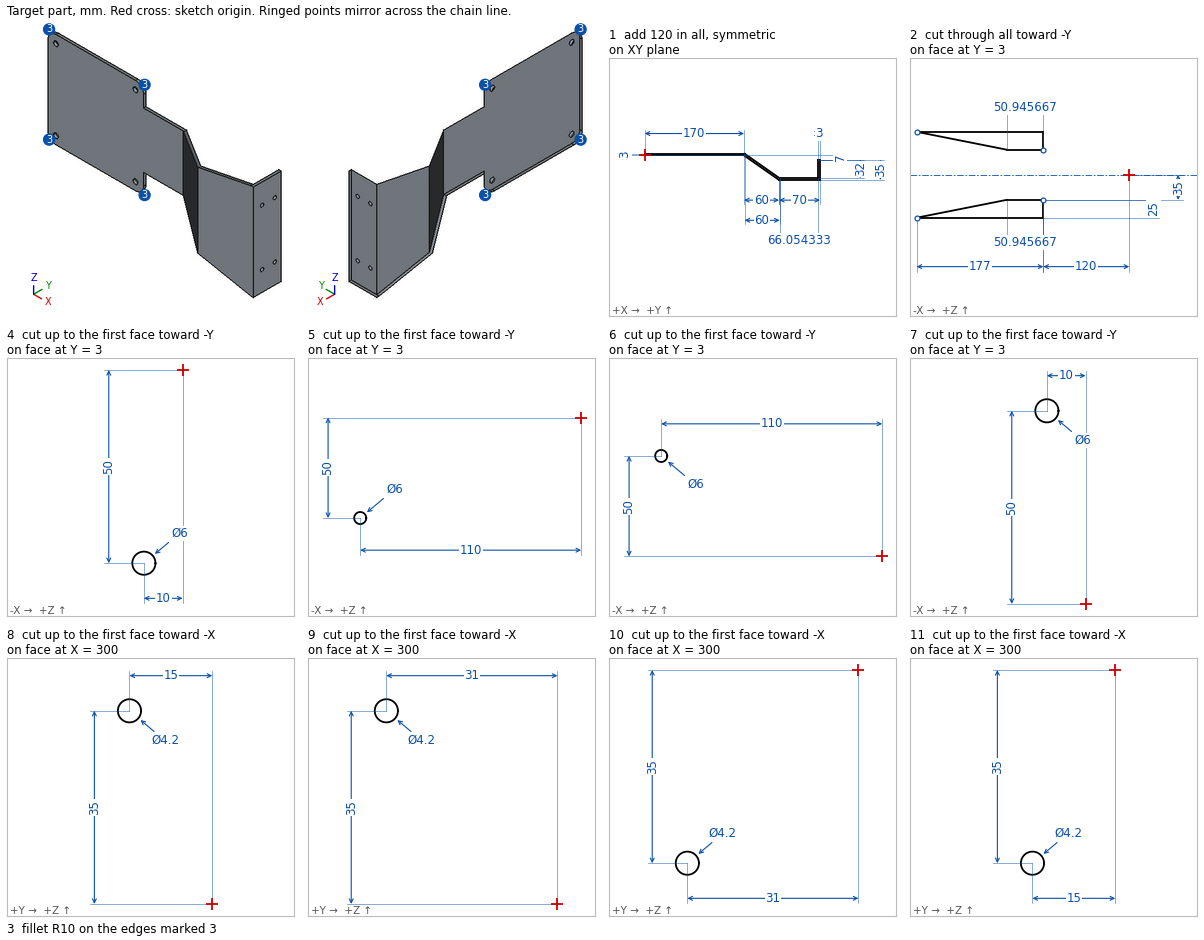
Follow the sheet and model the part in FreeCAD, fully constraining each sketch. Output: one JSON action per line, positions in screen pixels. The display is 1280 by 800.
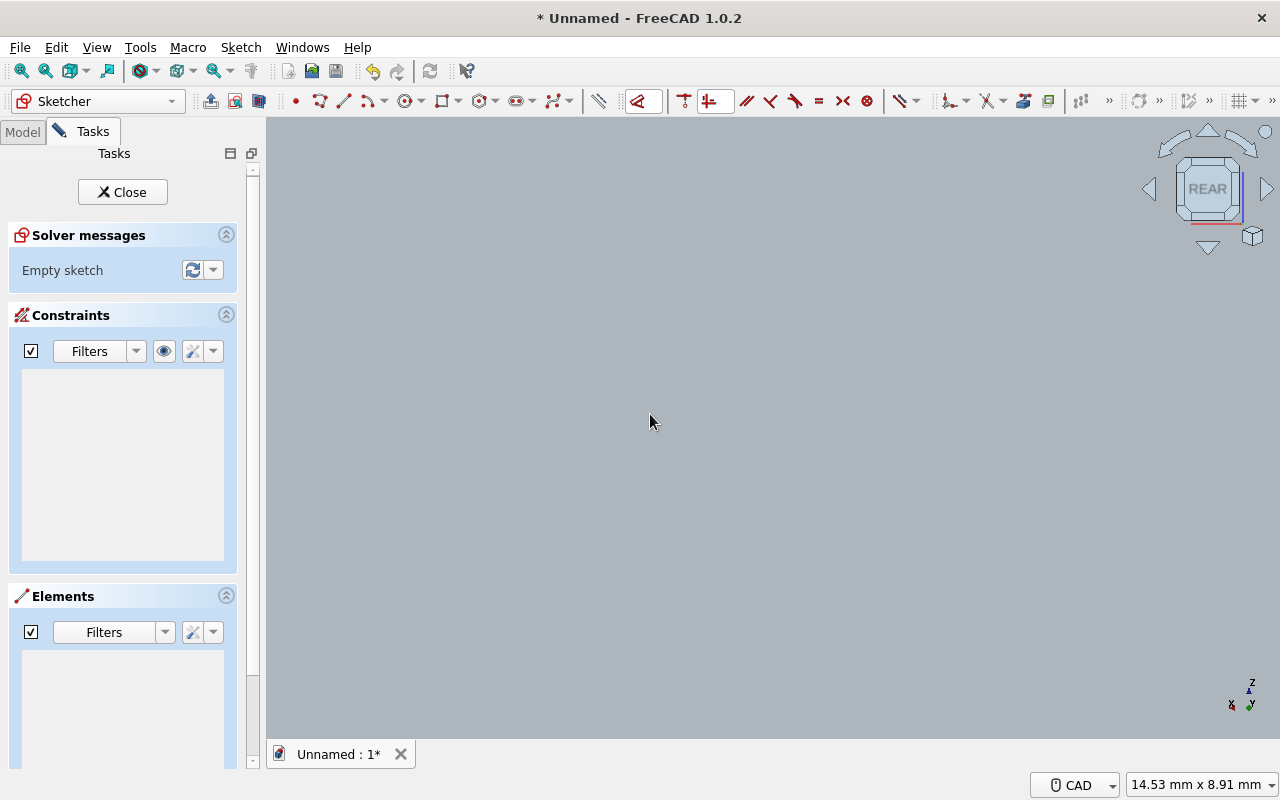
{"action": "left_click", "coordinate": [406, 102]}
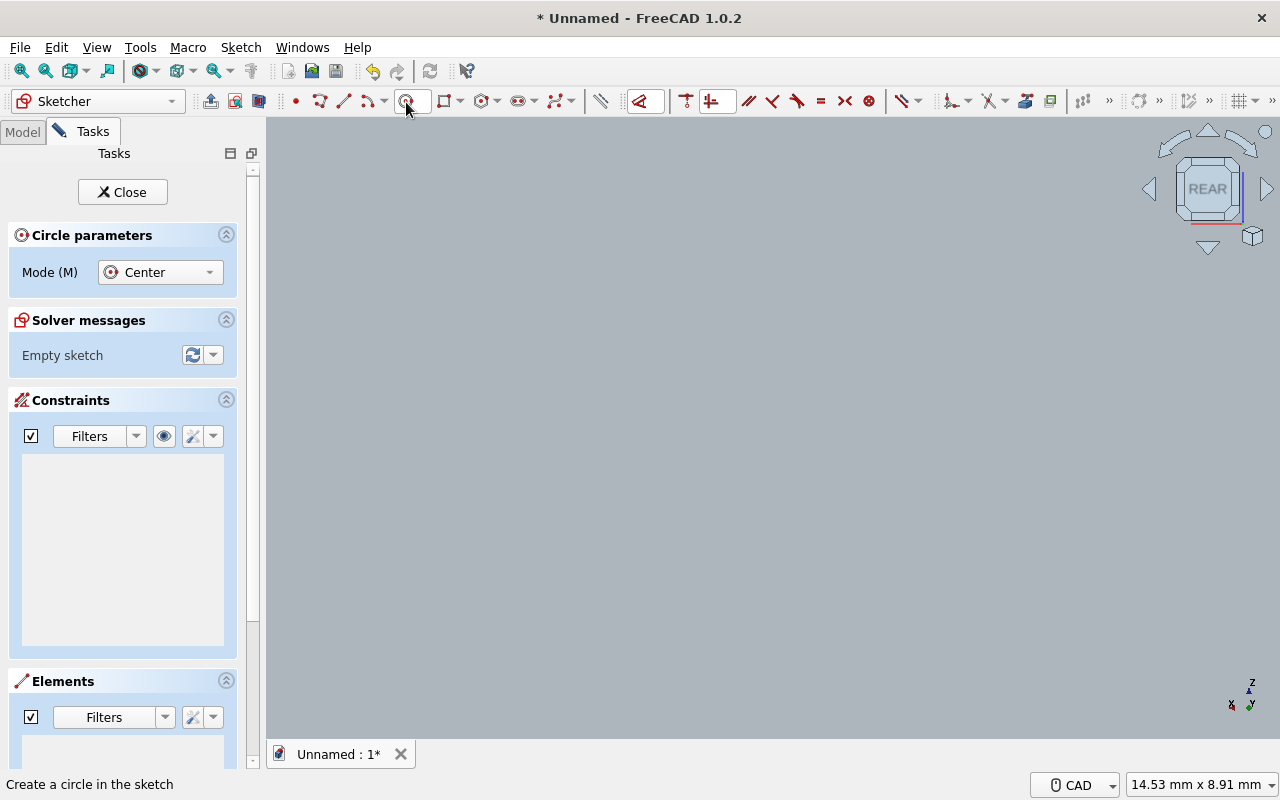
{"action": "left_click", "coordinate": [705, 427]}
{"action": "left_click", "coordinate": [853, 279]}
{"action": "key", "text": "Escape"}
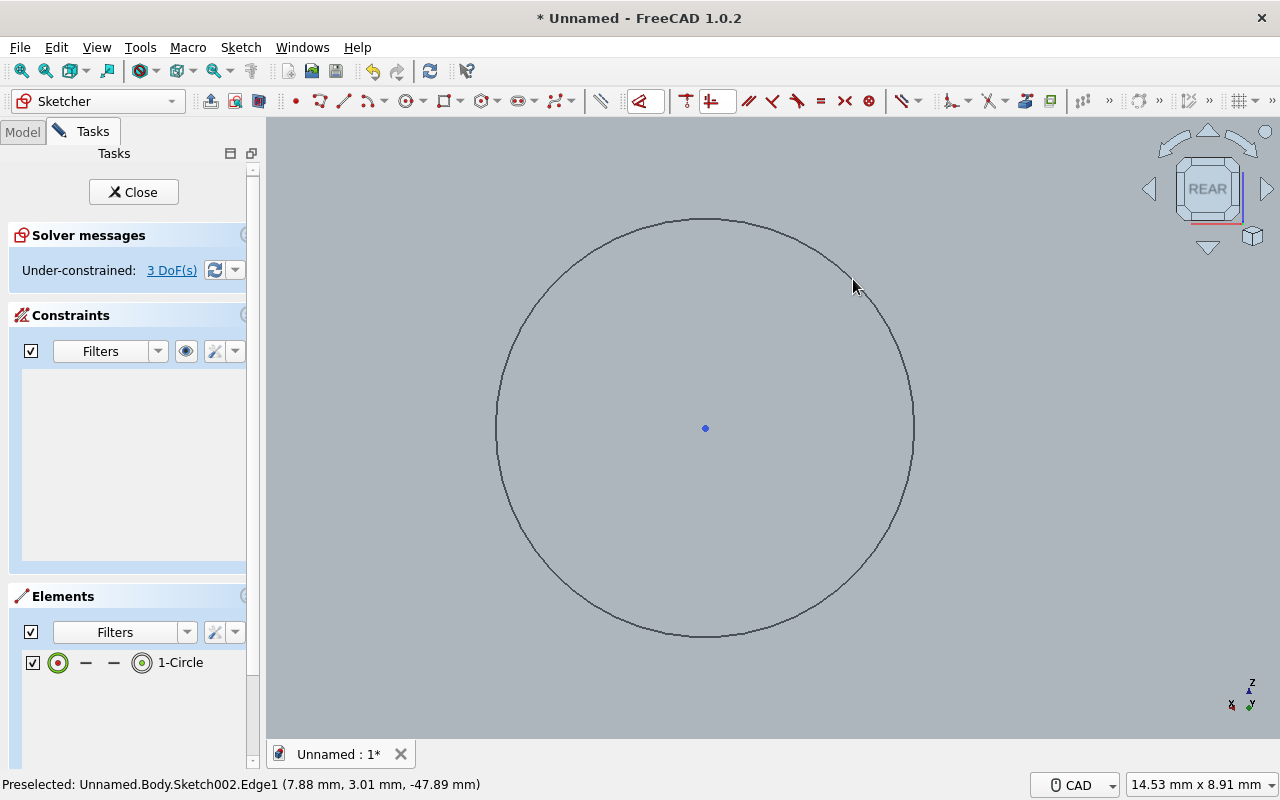
{"action": "left_click", "coordinate": [853, 280]}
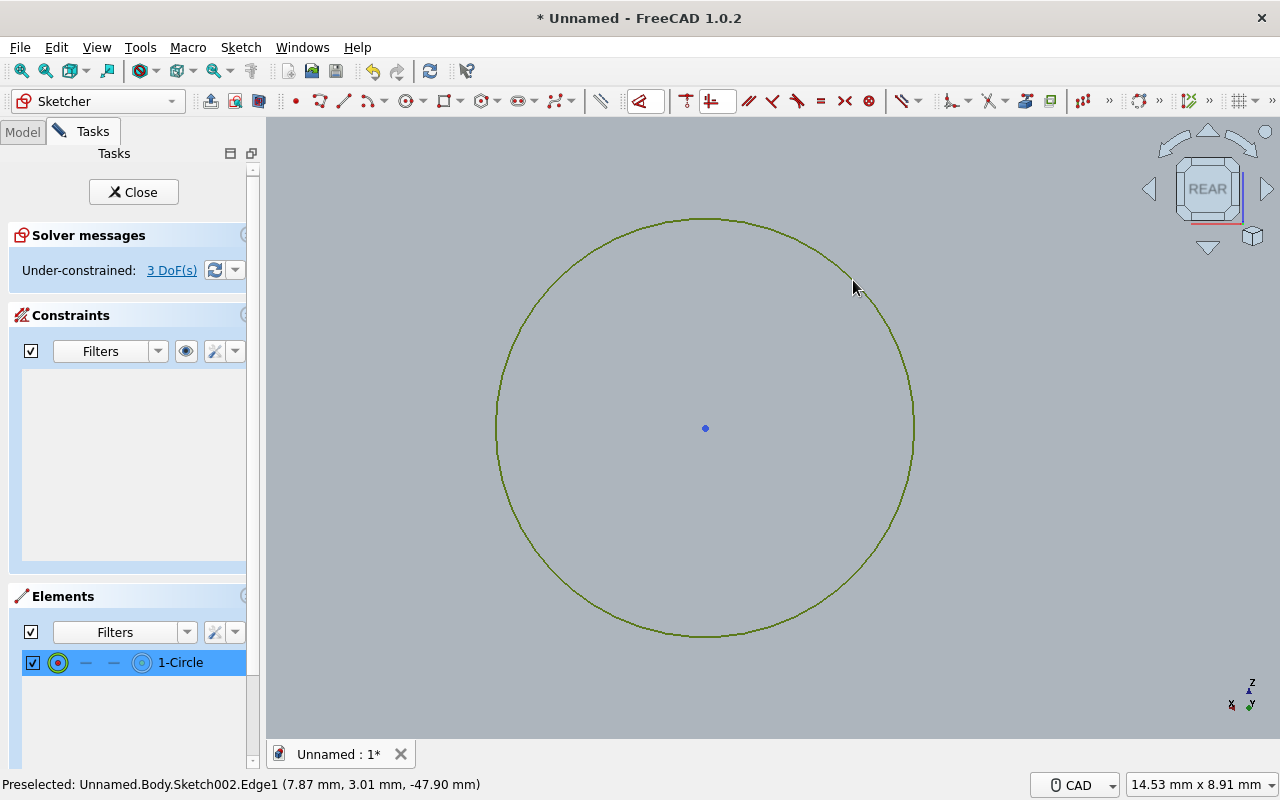
{"action": "key", "text": "k o"}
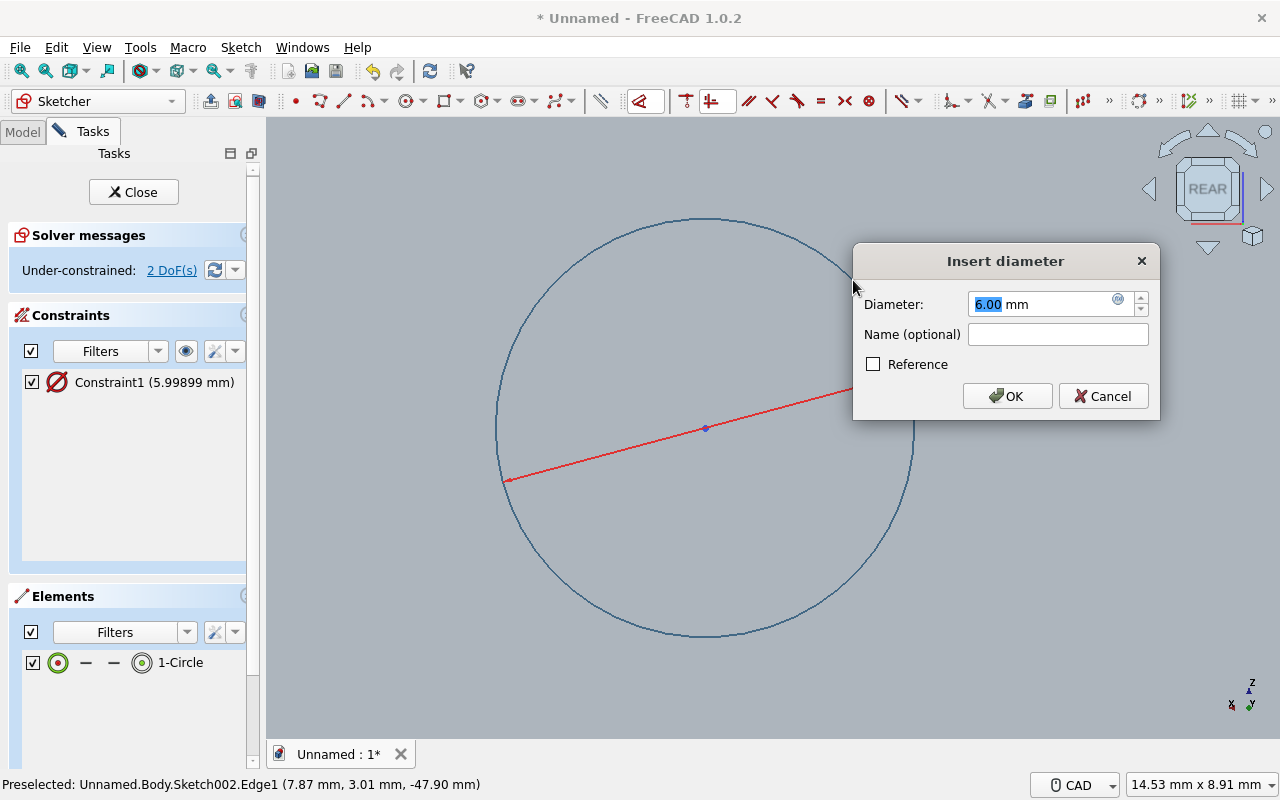
{"action": "type", "text": "6"}
{"action": "key", "text": "Return"}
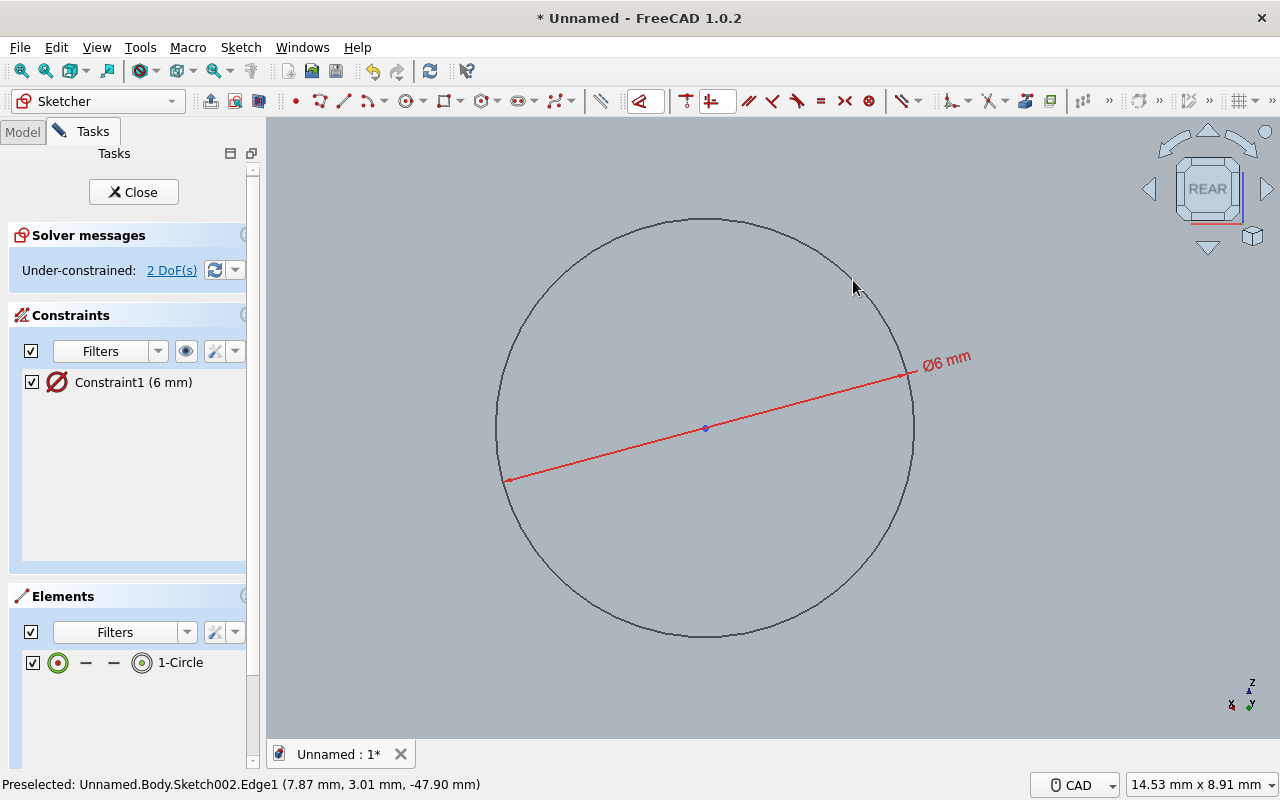
{"action": "left_click", "coordinate": [705, 428]}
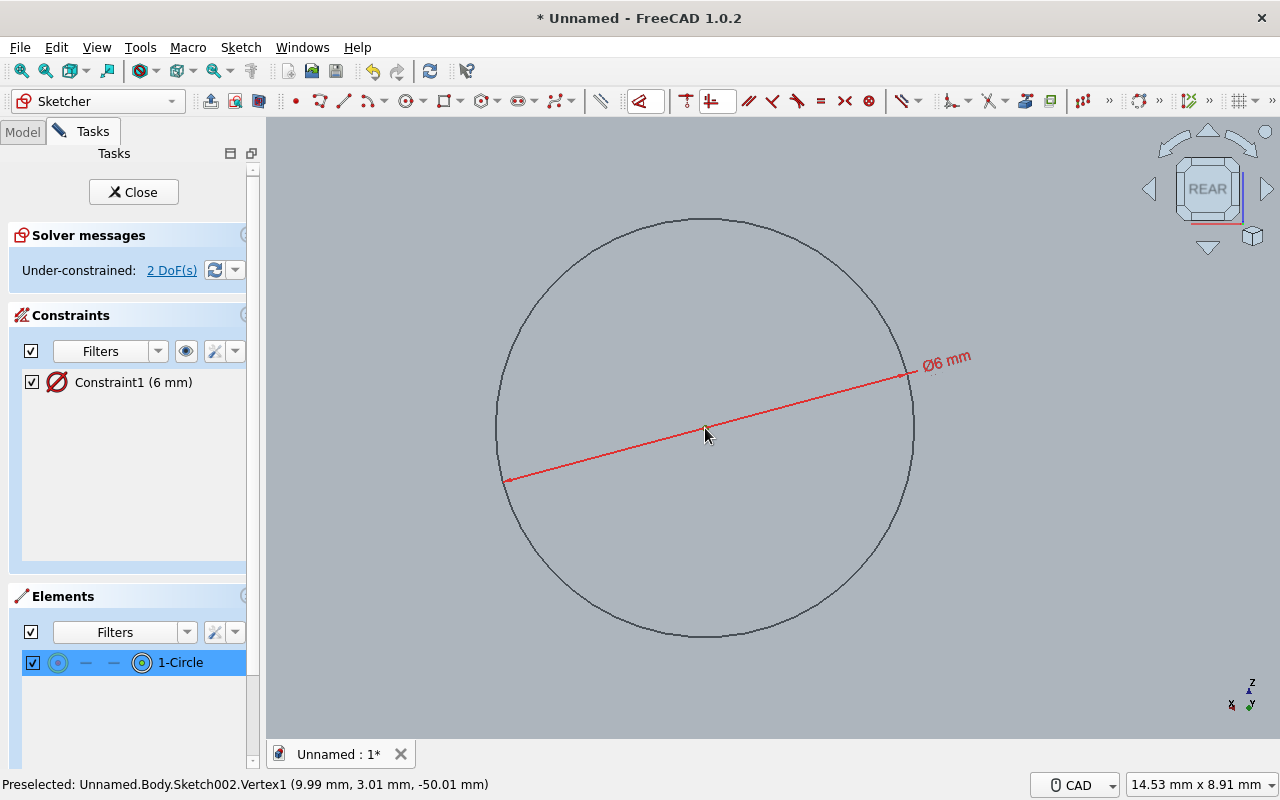
{"action": "key", "text": "l"}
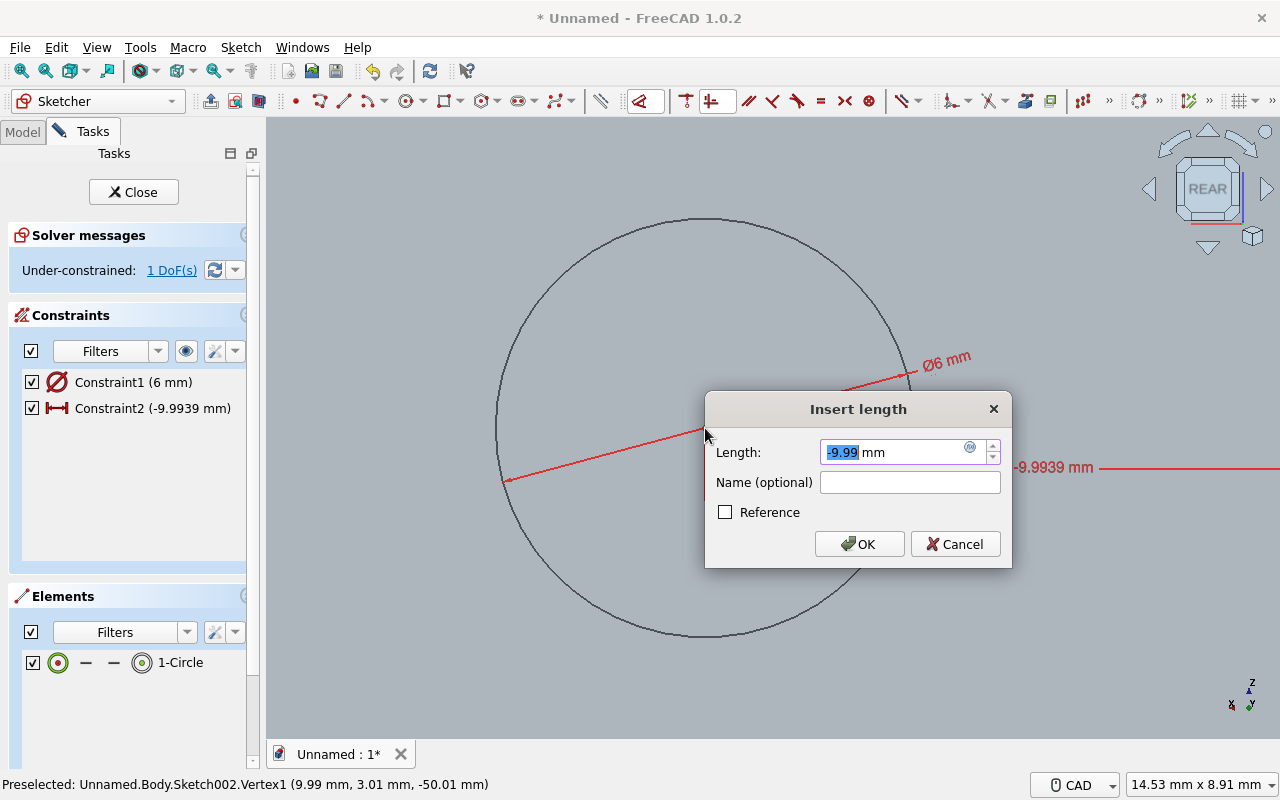
{"action": "type", "text": "-10"}
{"action": "key", "text": "Return"}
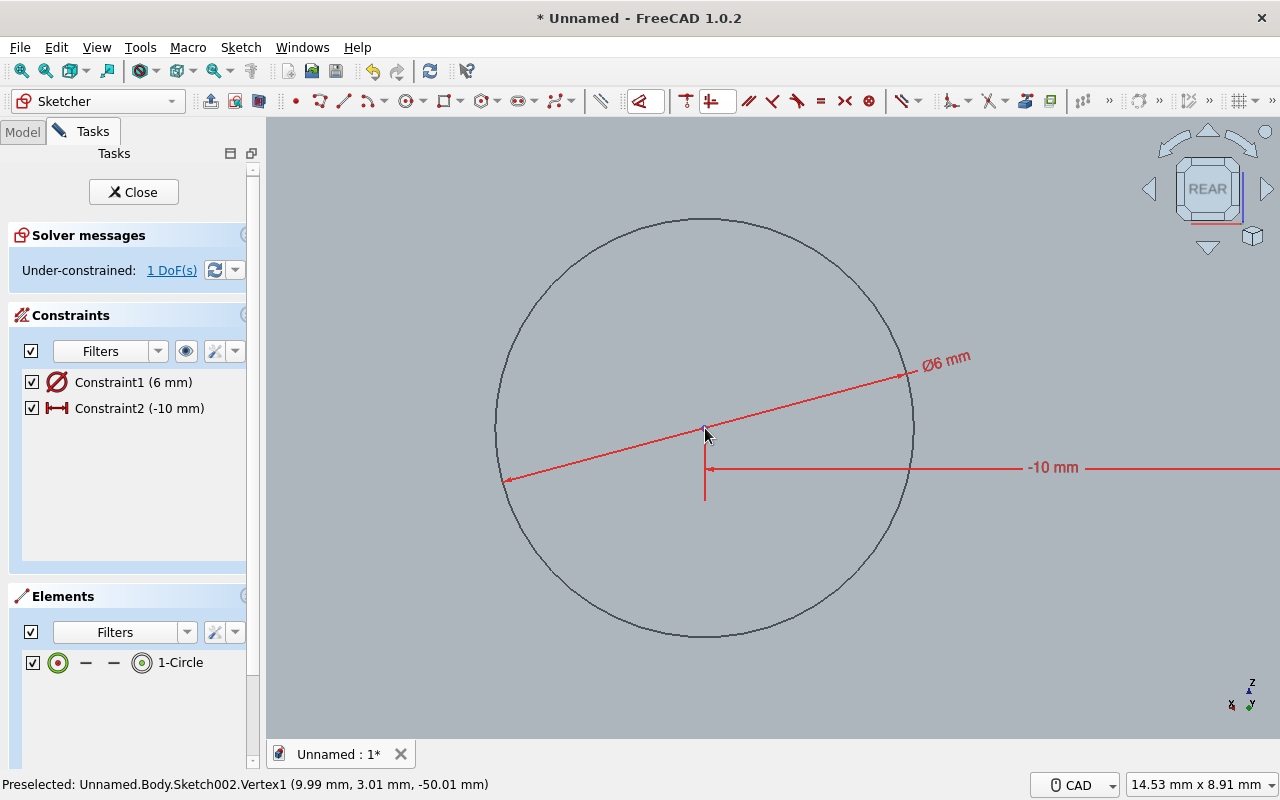
{"action": "left_click", "coordinate": [705, 428]}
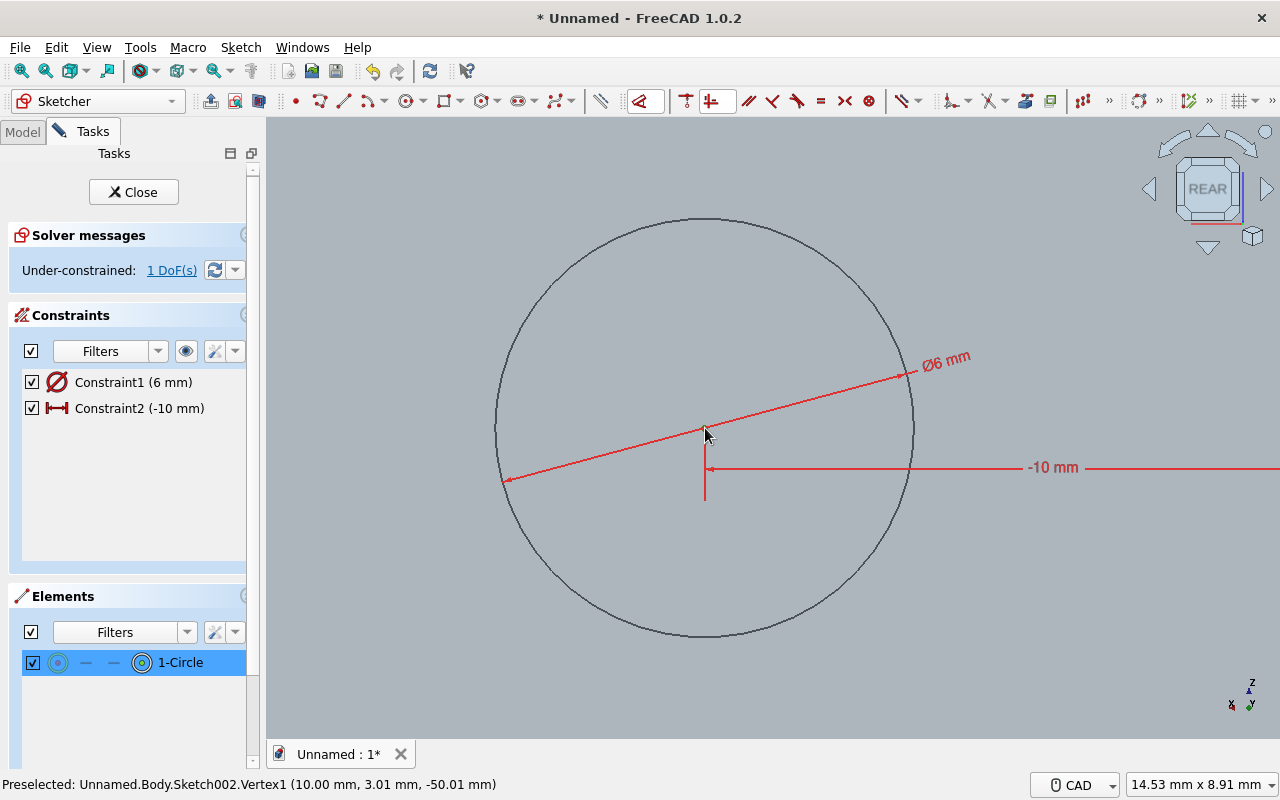
{"action": "left_click", "coordinate": [658, 102]}